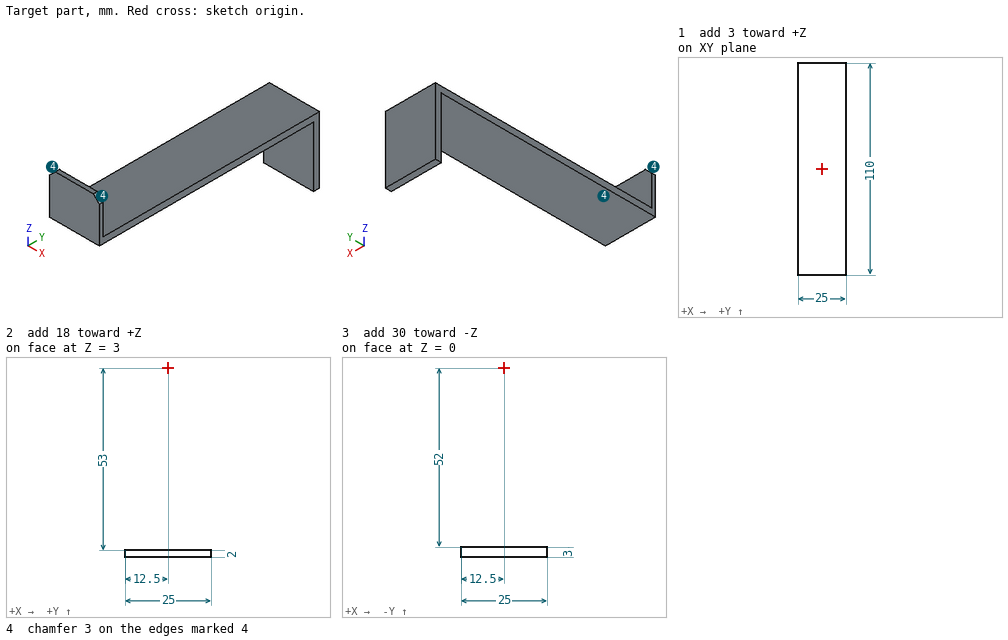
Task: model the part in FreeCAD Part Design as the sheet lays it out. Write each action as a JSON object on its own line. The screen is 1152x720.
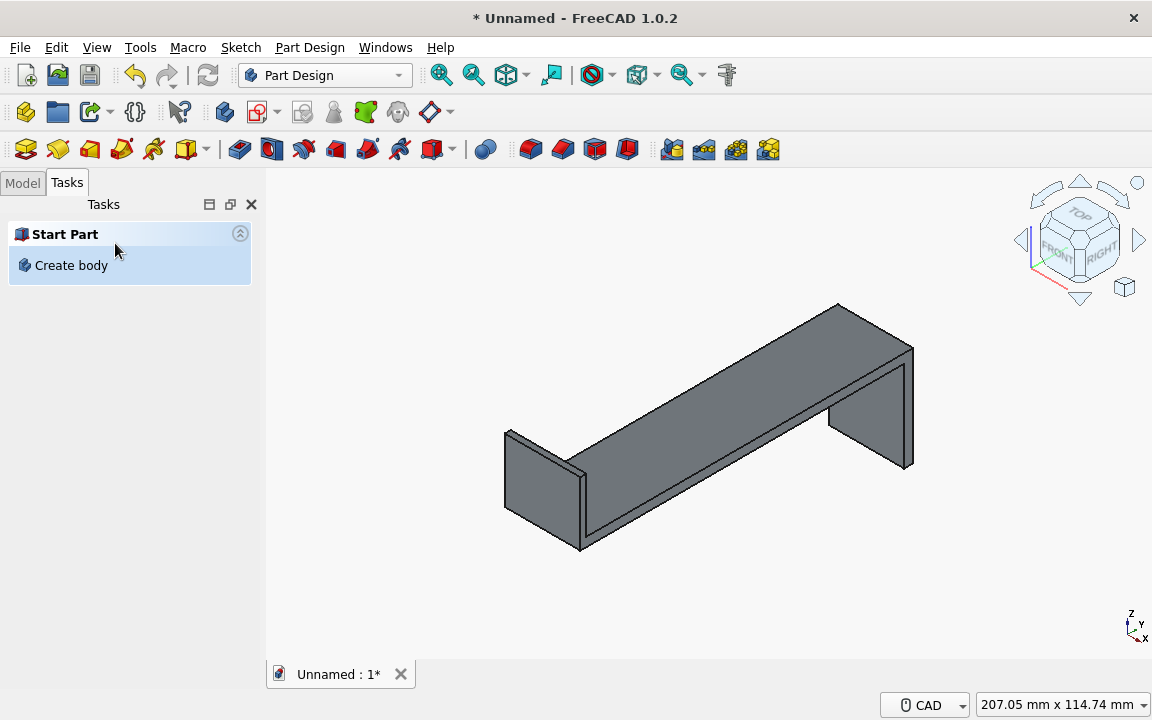
{"action": "scroll", "coordinate": [508, 431], "scroll_direction": "up", "scroll_amount": 8}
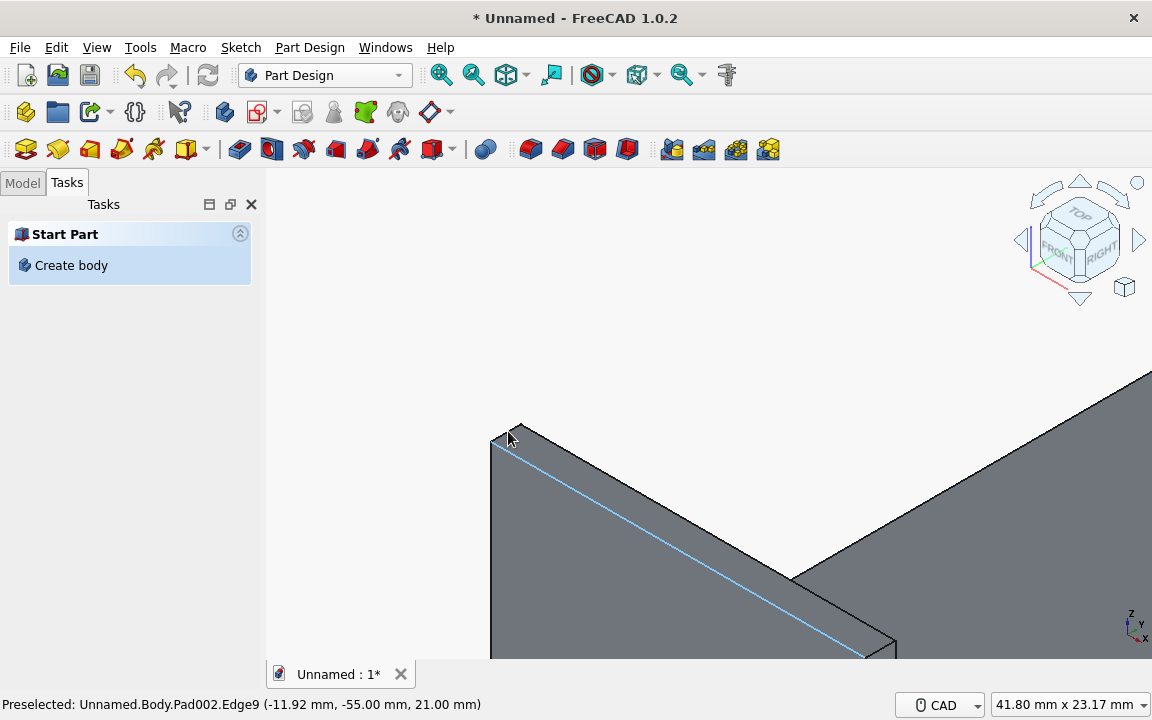
{"action": "key", "text": "v f"}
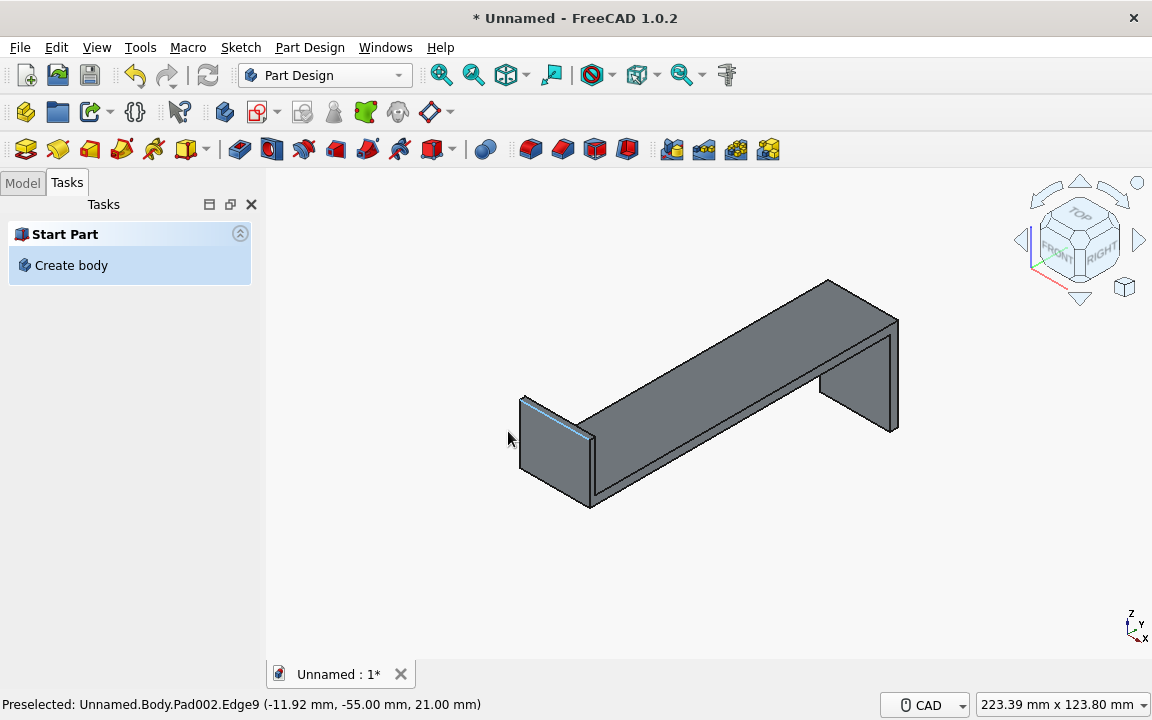
{"action": "key", "text": "2"}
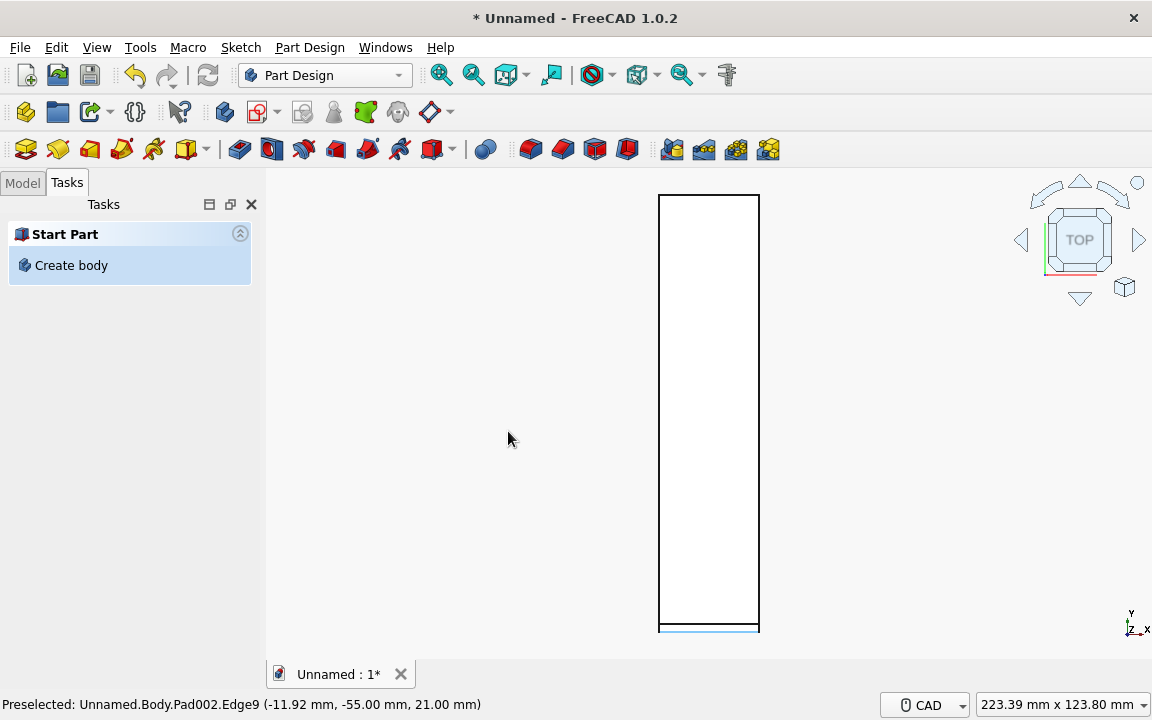
{"action": "scroll", "coordinate": [659, 627], "scroll_direction": "up", "scroll_amount": 9}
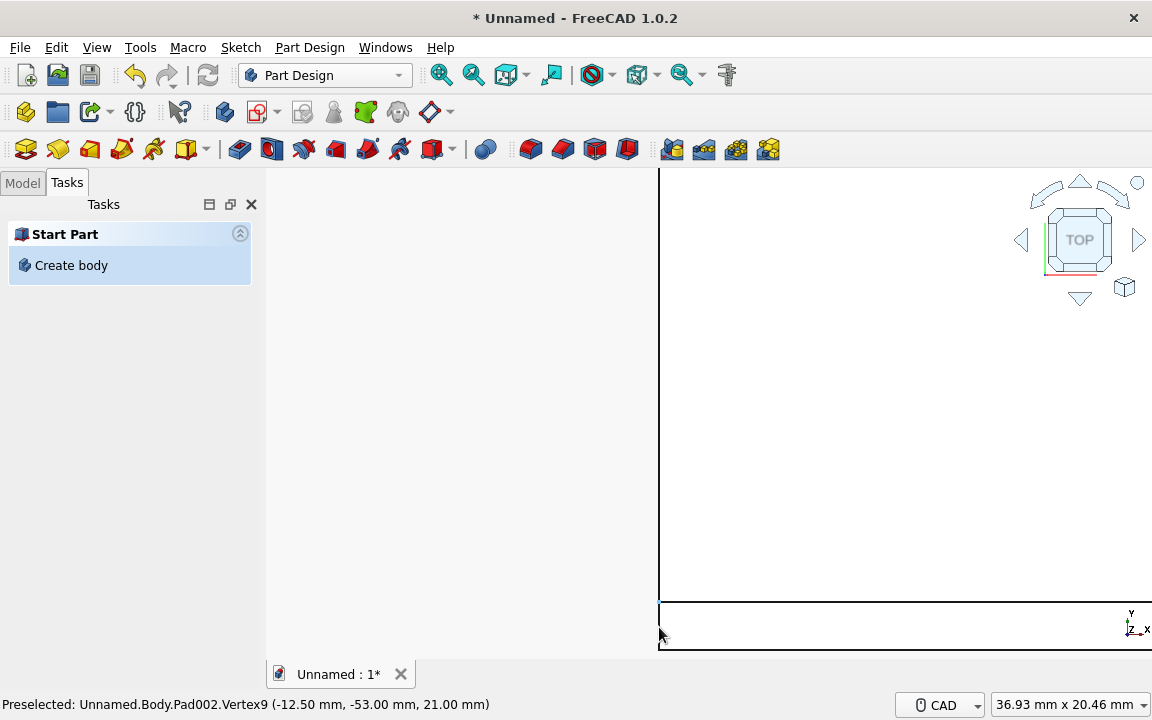
{"action": "left_click", "coordinate": [659, 625]}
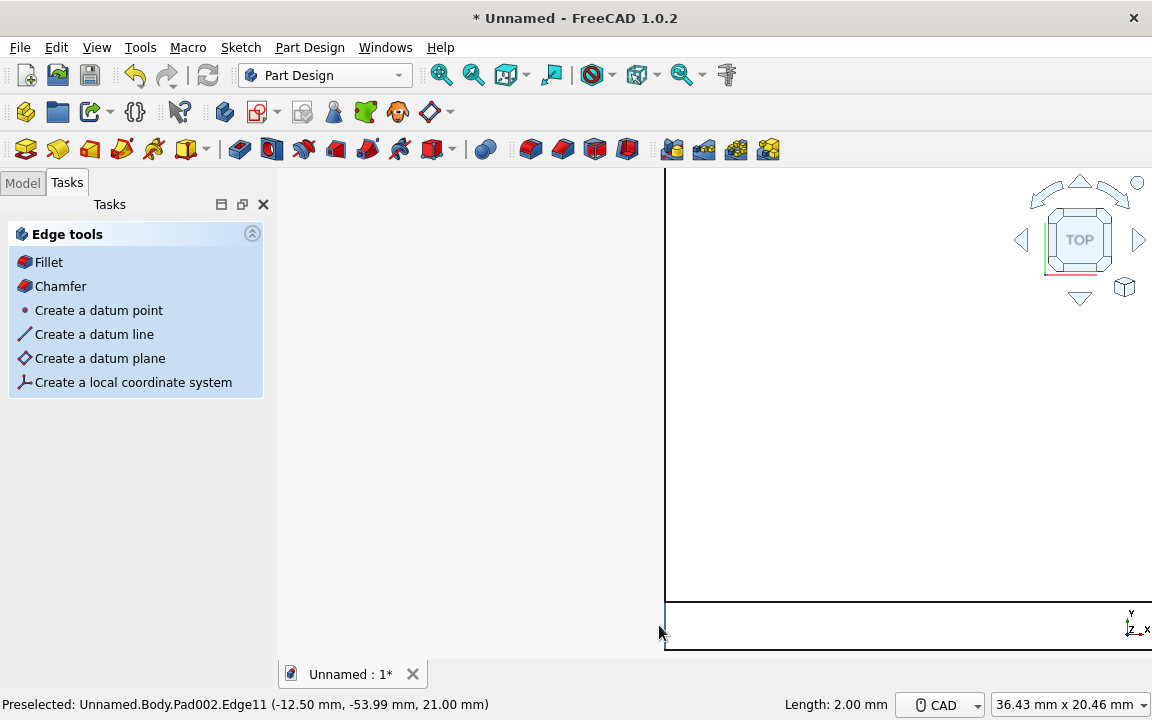
{"action": "key", "text": "v f"}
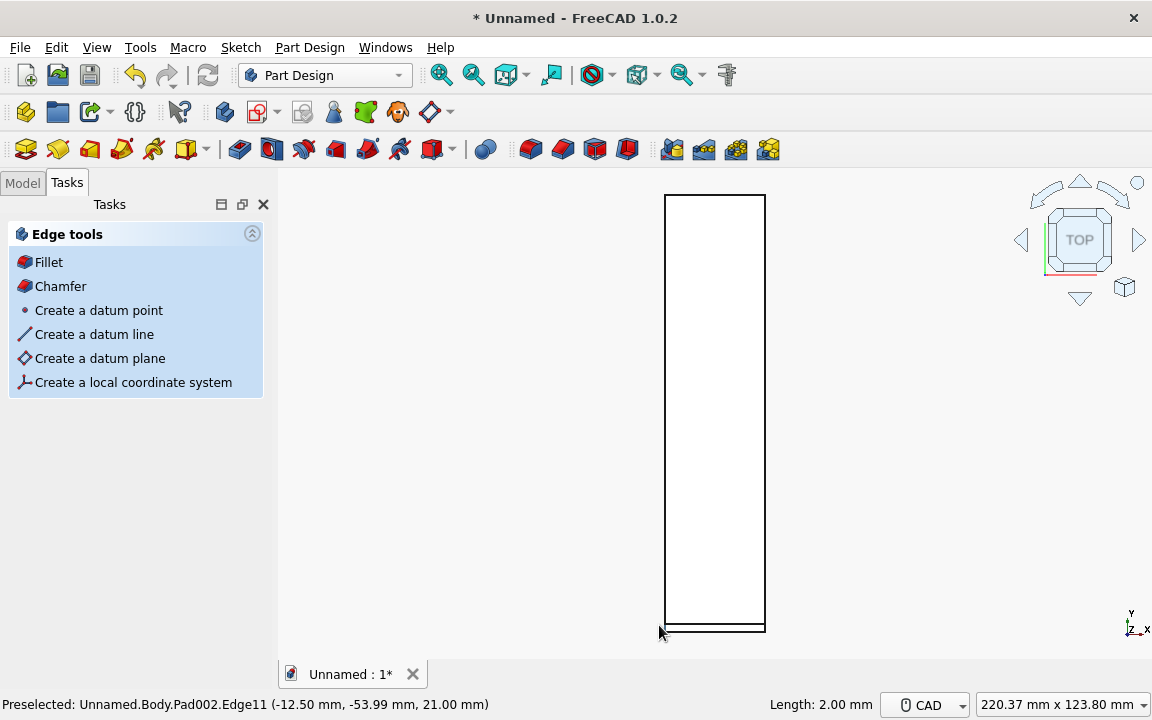
{"action": "key", "text": "1"}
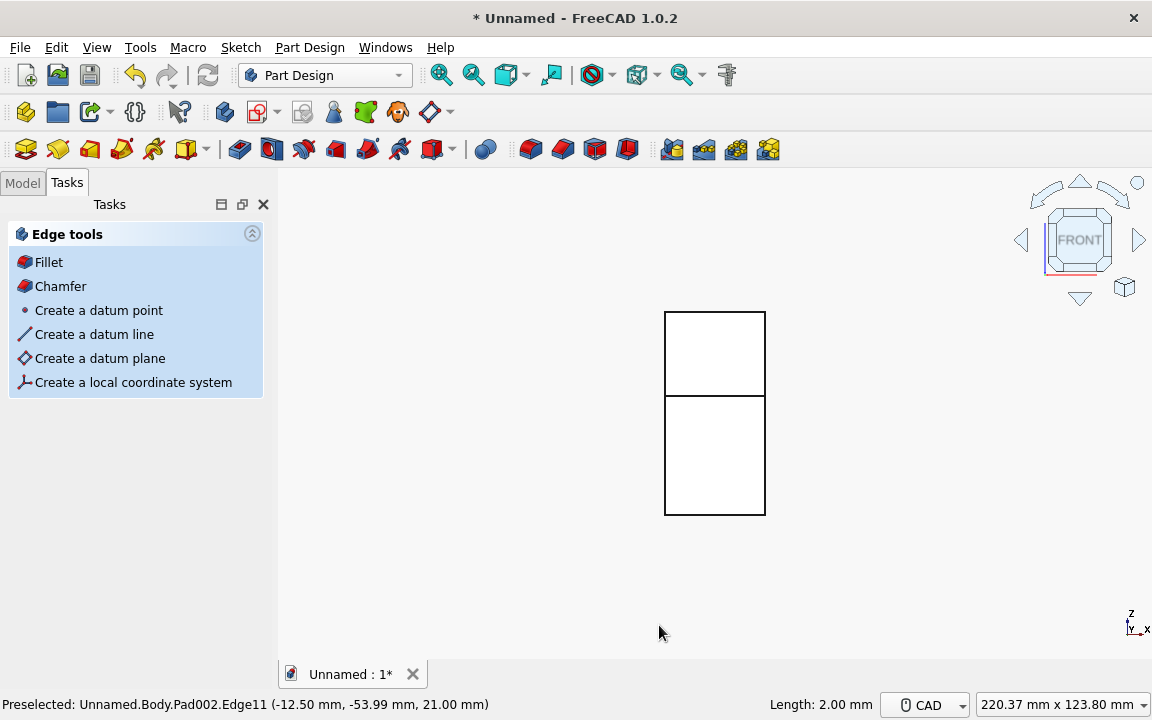
{"action": "left_click", "coordinate": [442, 76]}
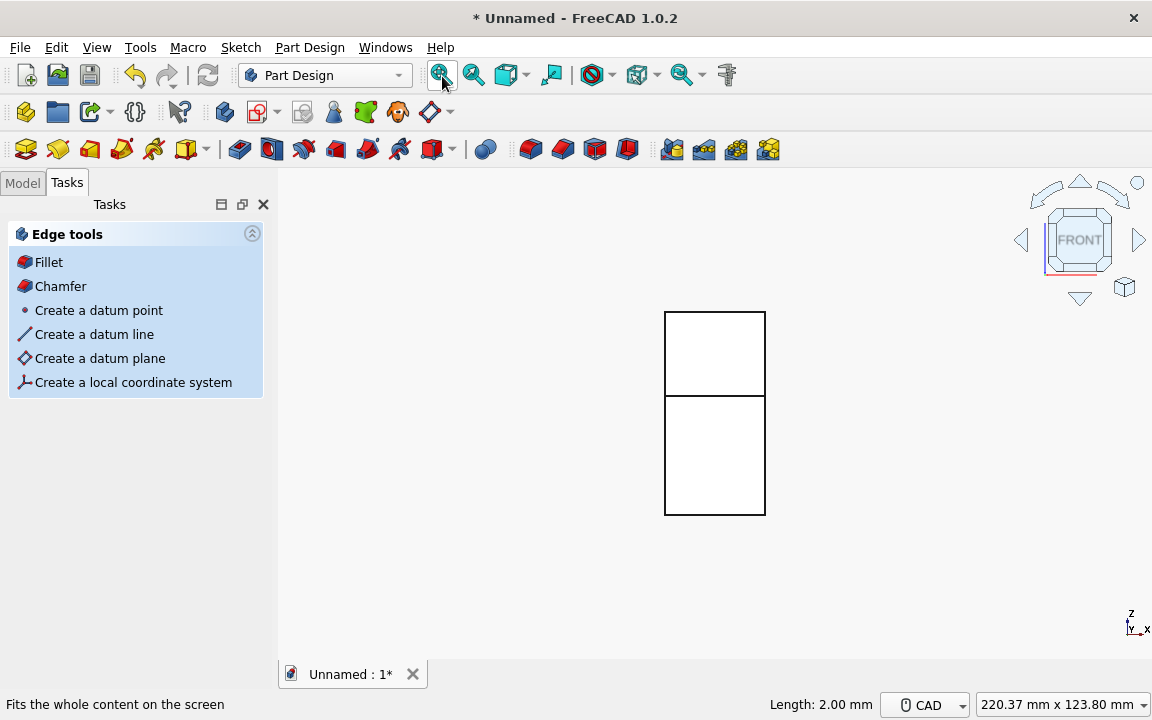
{"action": "scroll", "coordinate": [765, 311], "scroll_direction": "up", "scroll_amount": 9}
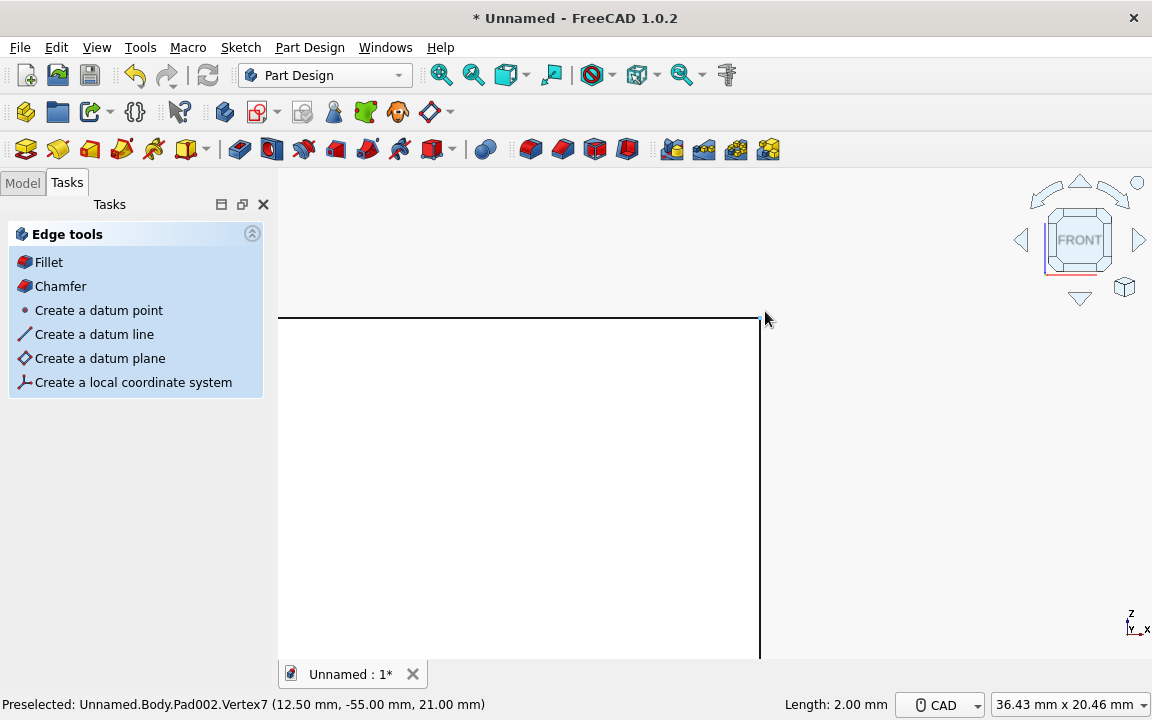
{"action": "key", "text": "v f"}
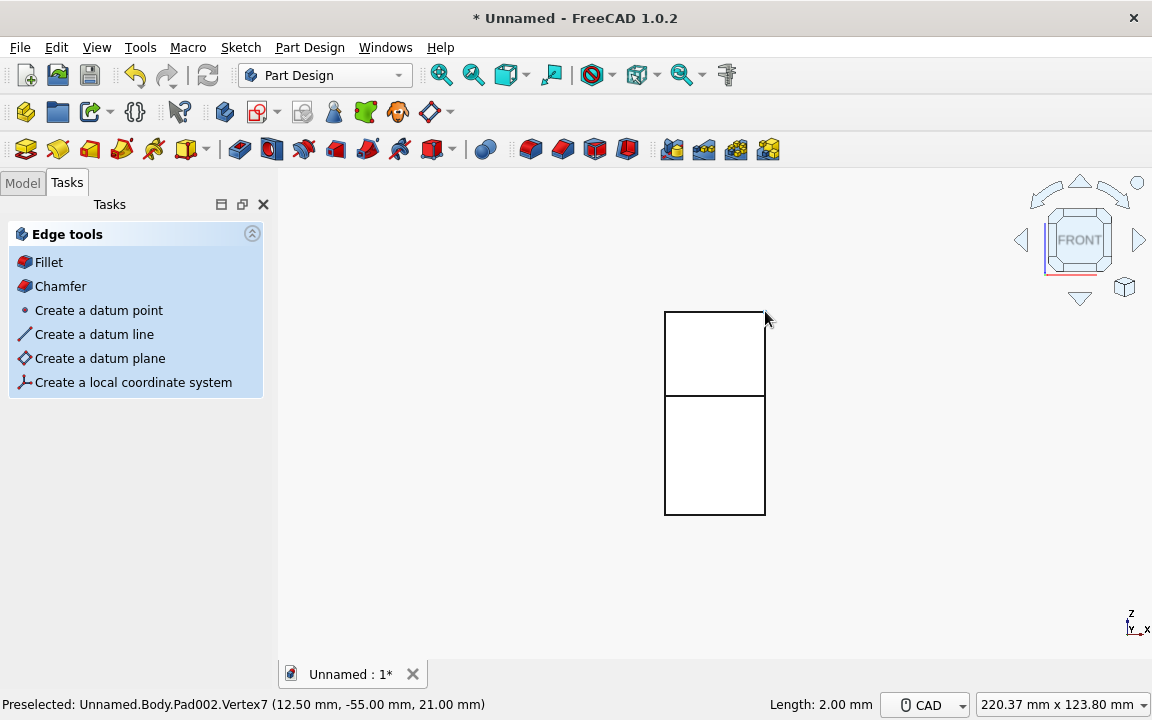
{"action": "key", "text": "3"}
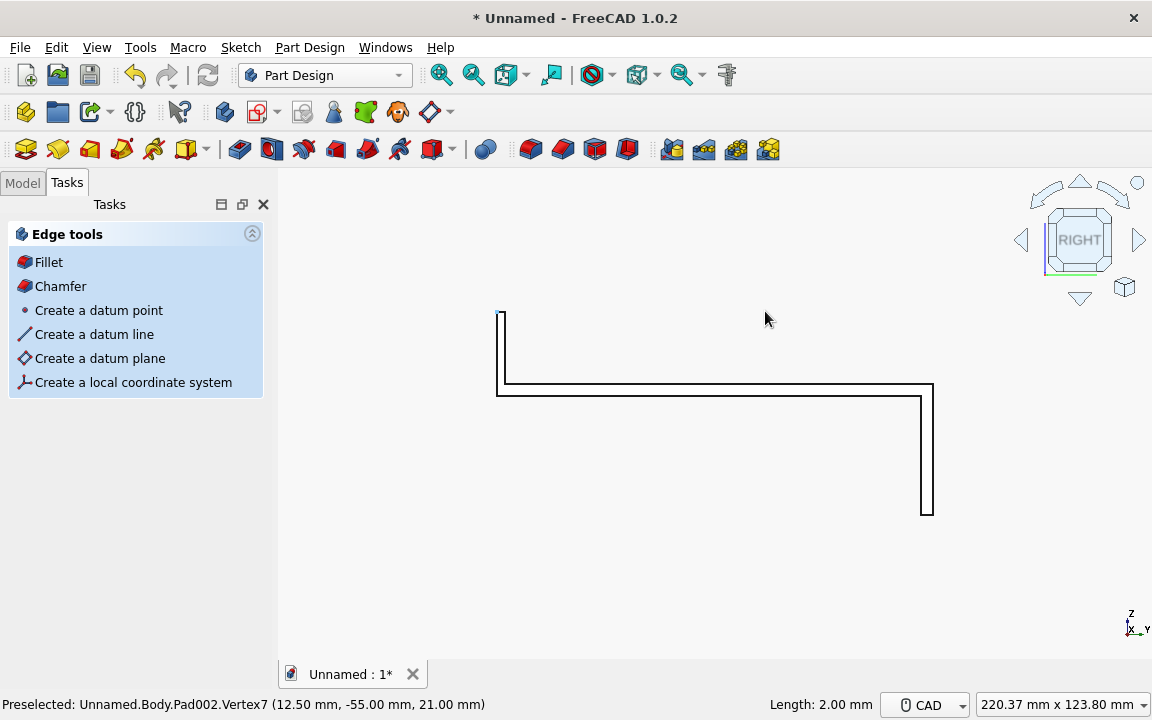
{"action": "scroll", "coordinate": [501, 311], "scroll_direction": "up", "scroll_amount": 9}